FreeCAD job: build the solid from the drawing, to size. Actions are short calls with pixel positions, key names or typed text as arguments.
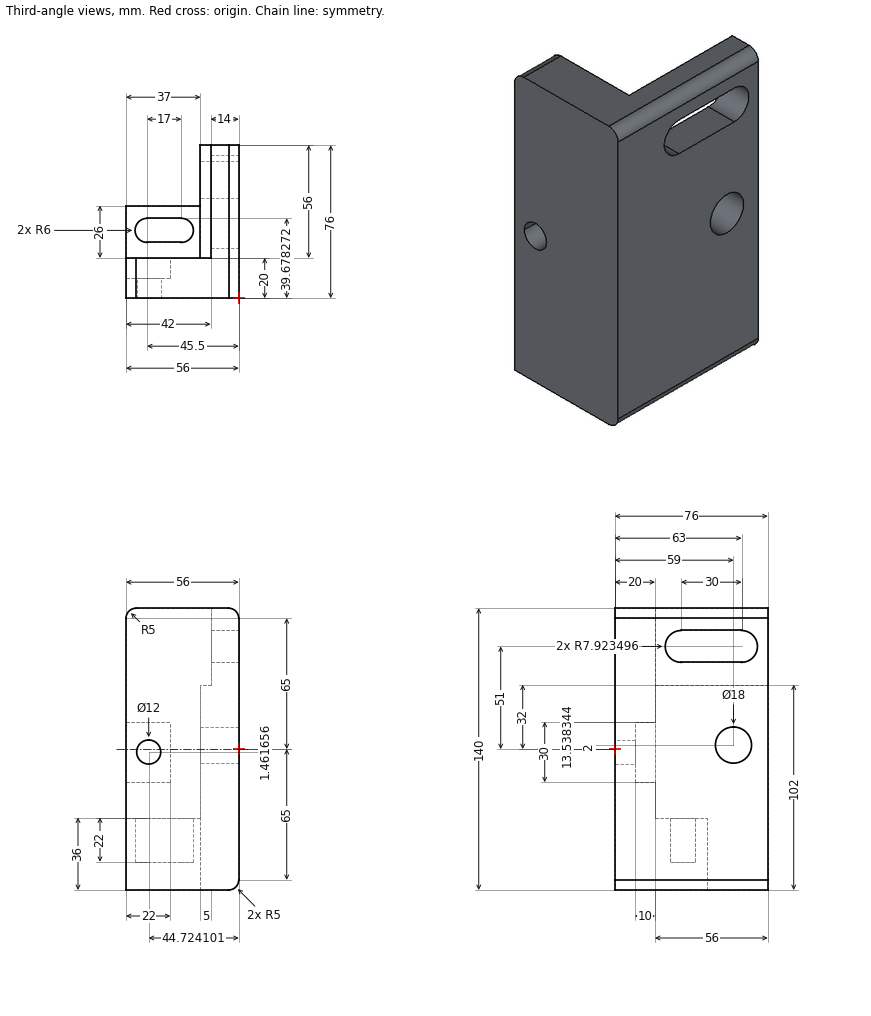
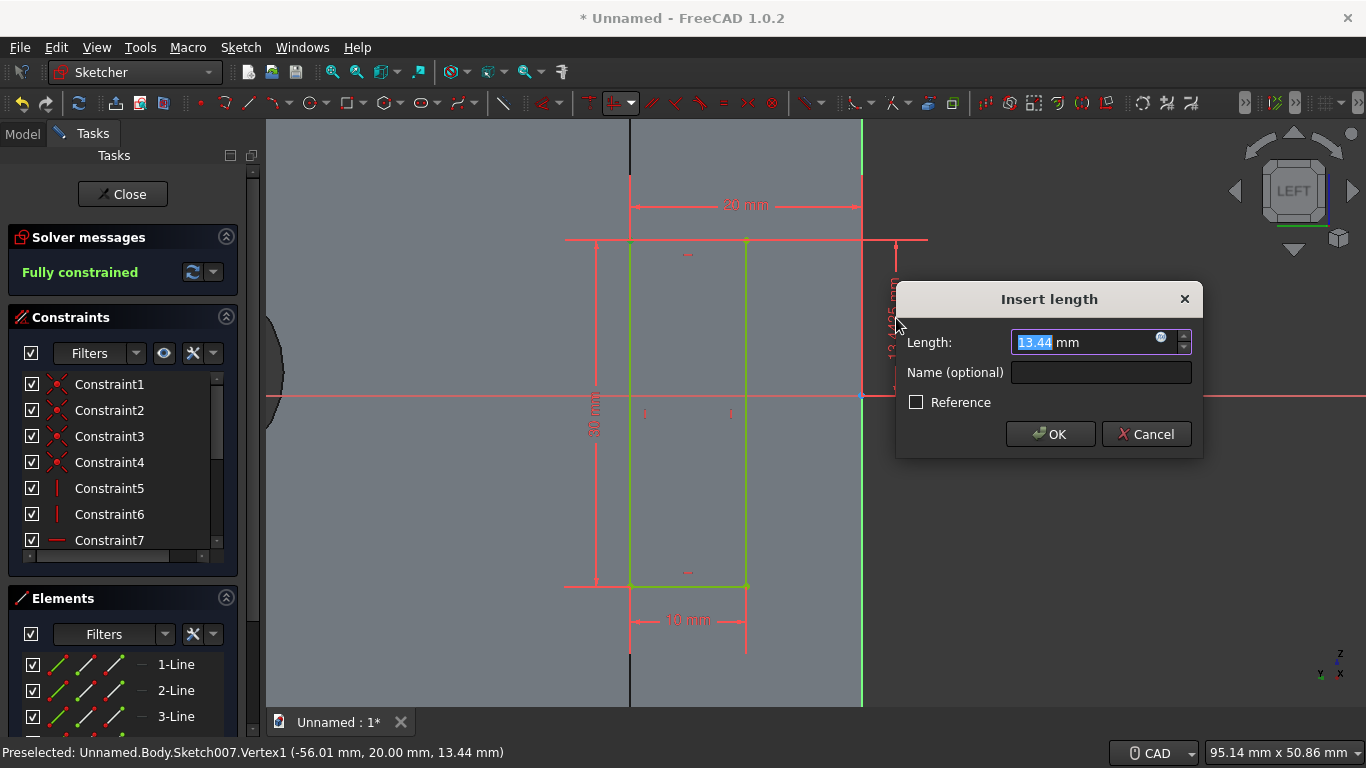
text(13.538344)
key(Return)
key(Escape)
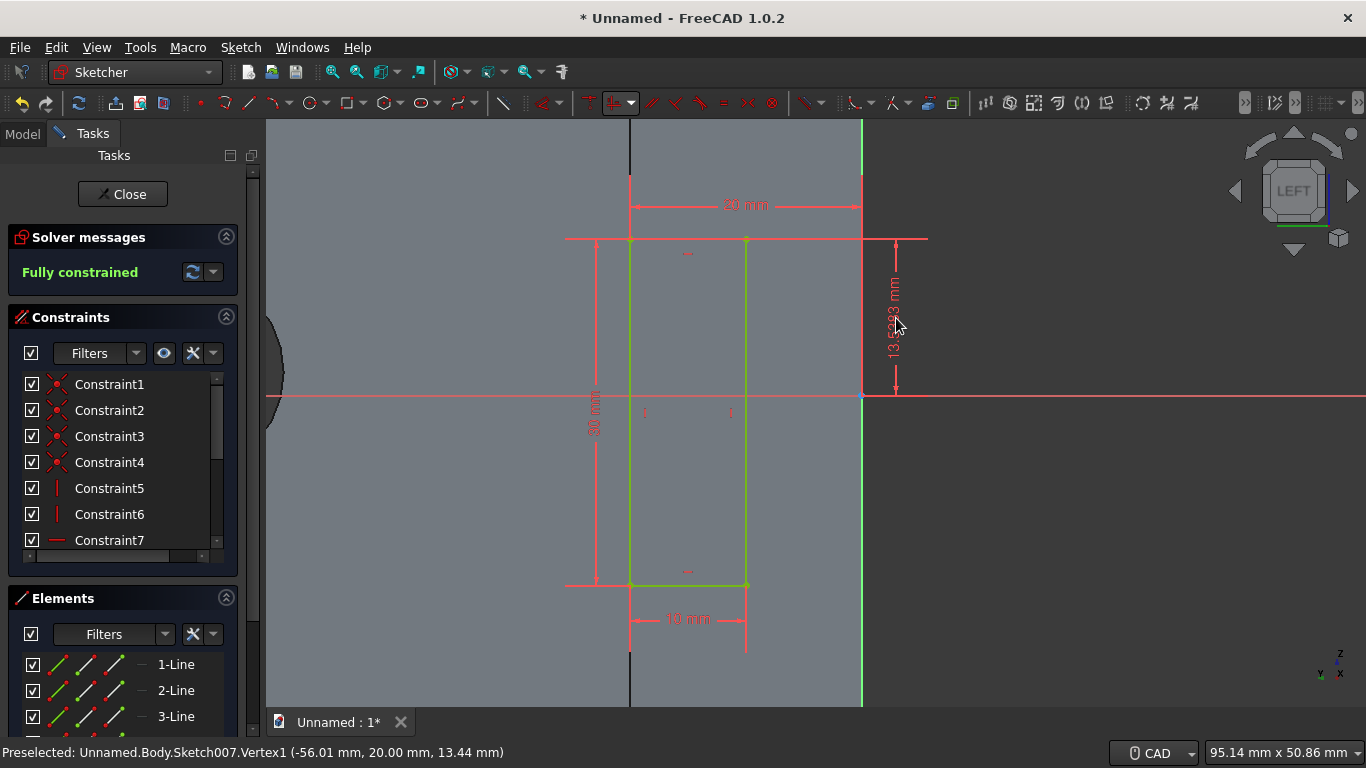
click(123, 194)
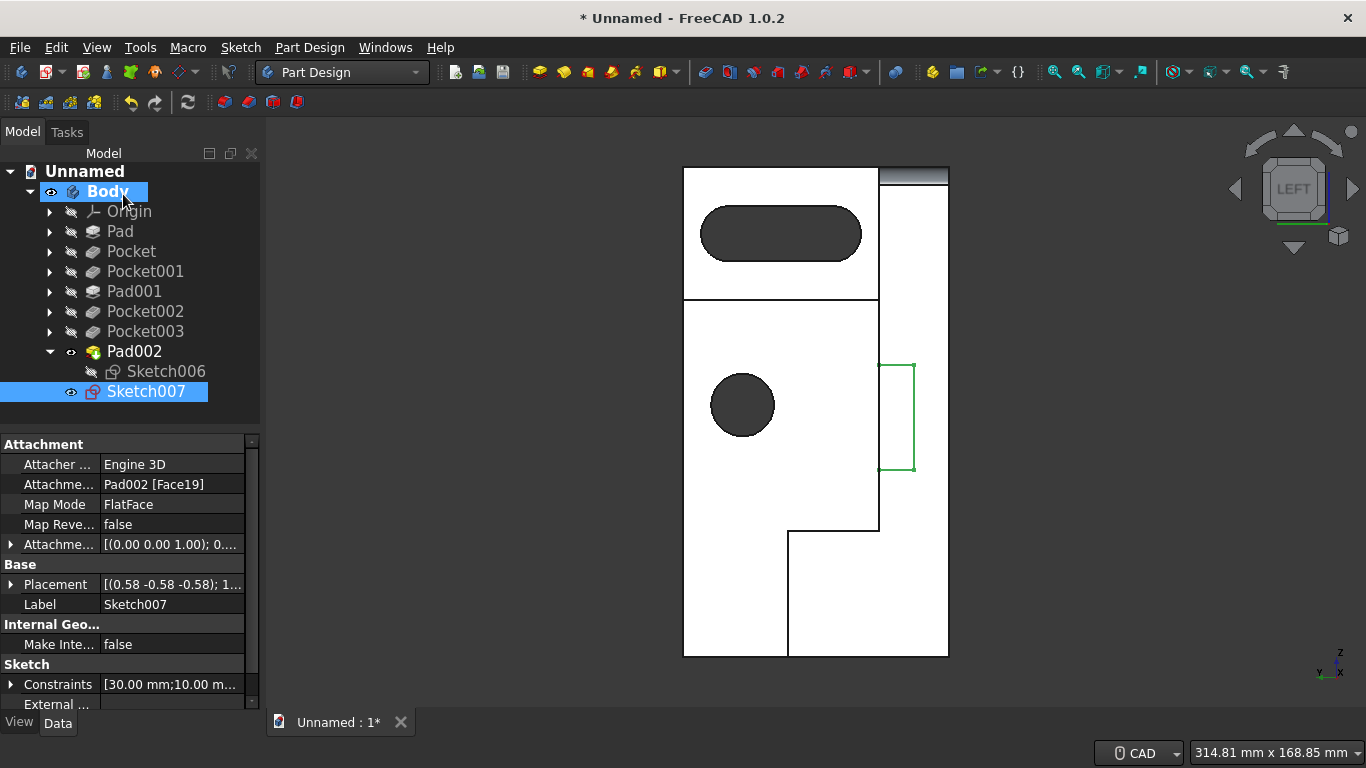
click(706, 72)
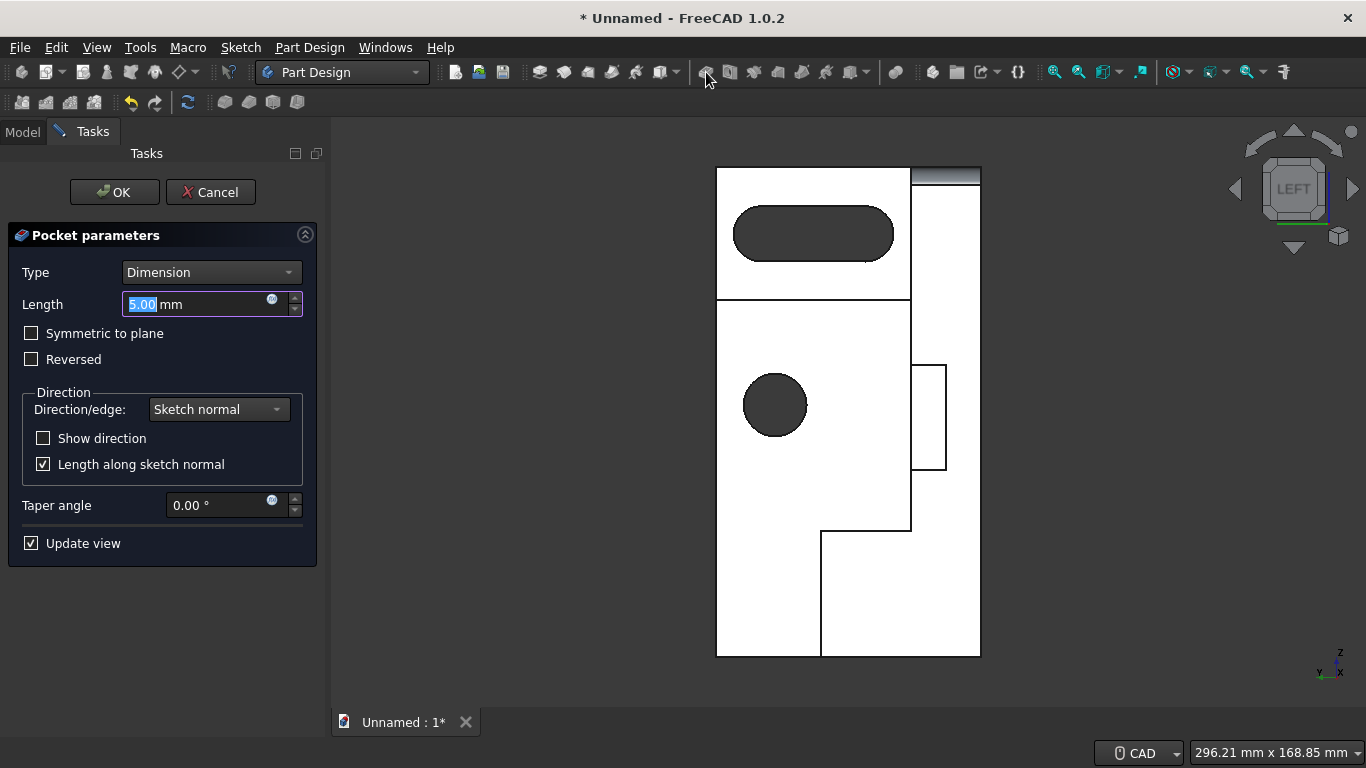
text(22)
key(Tab)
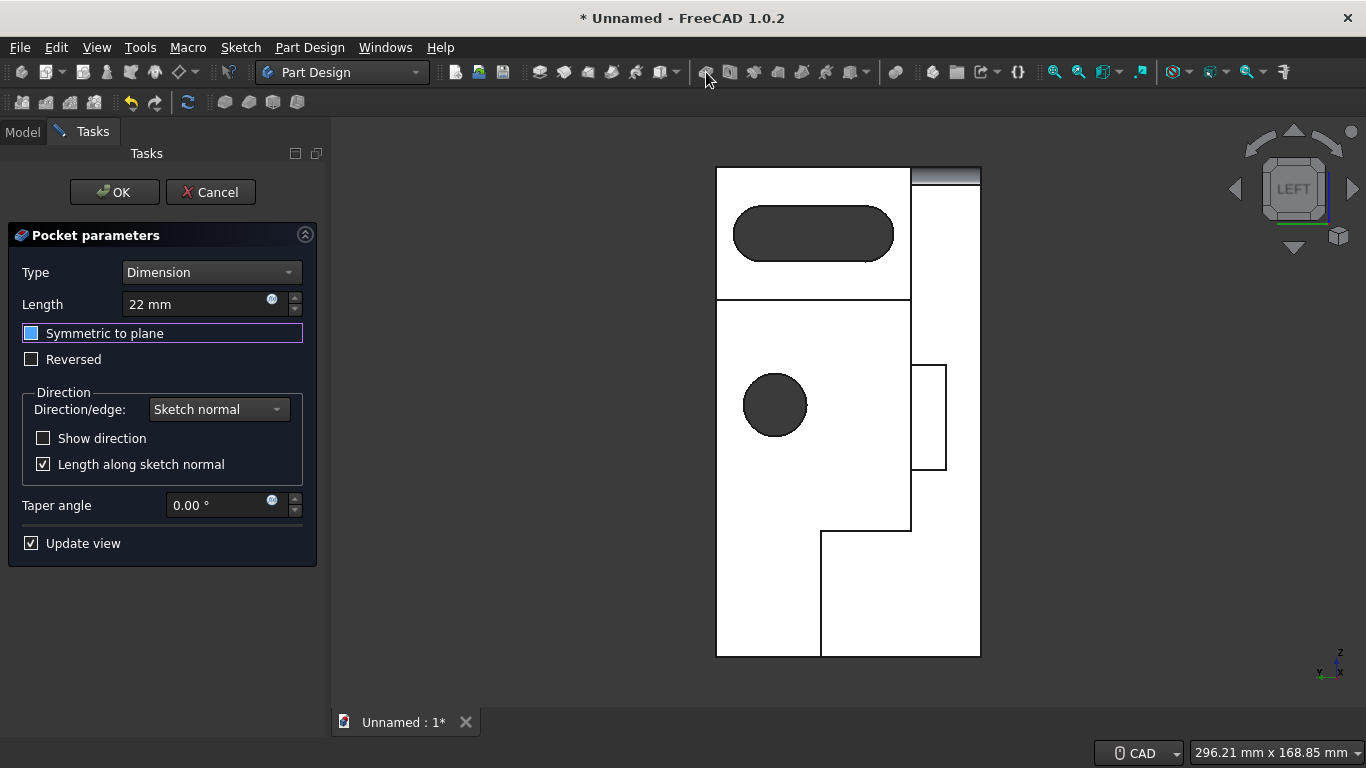
click(115, 192)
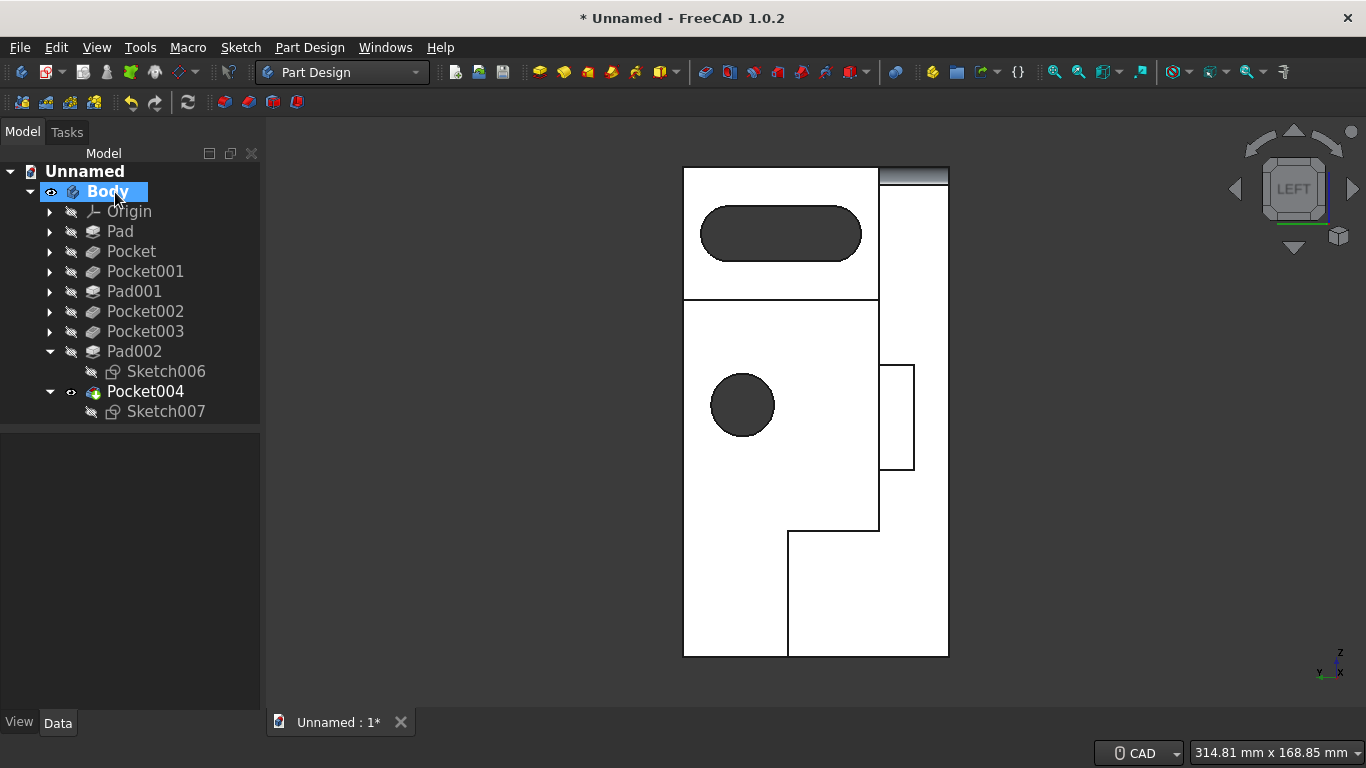
key(4)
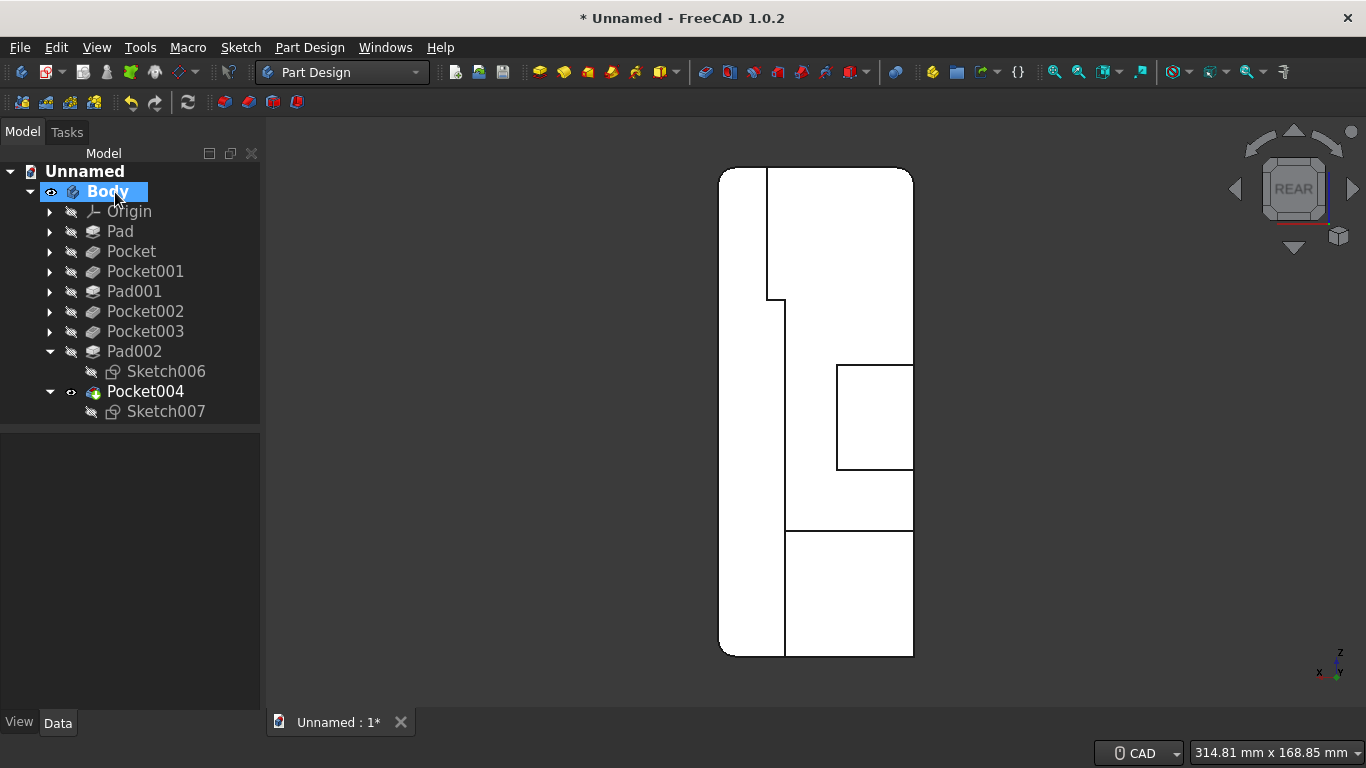
click(875, 416)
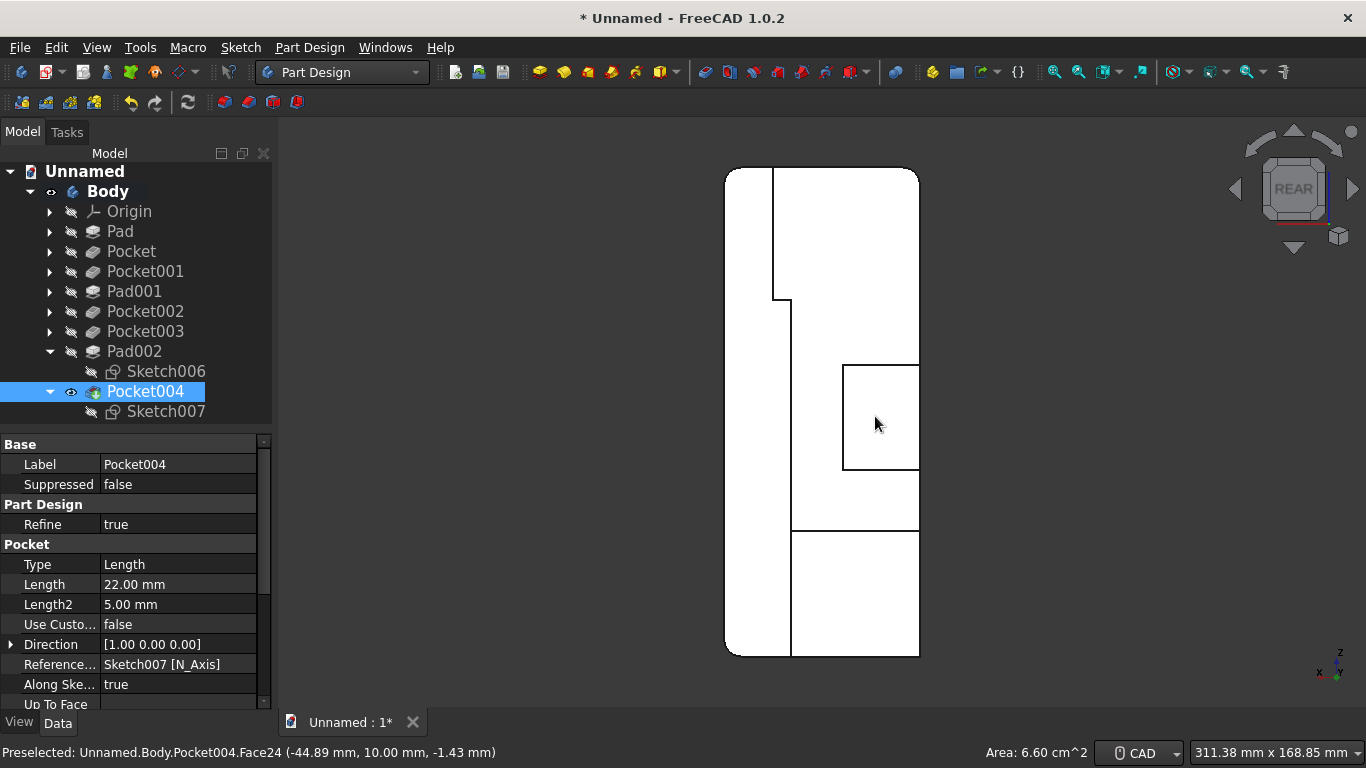
click(46, 72)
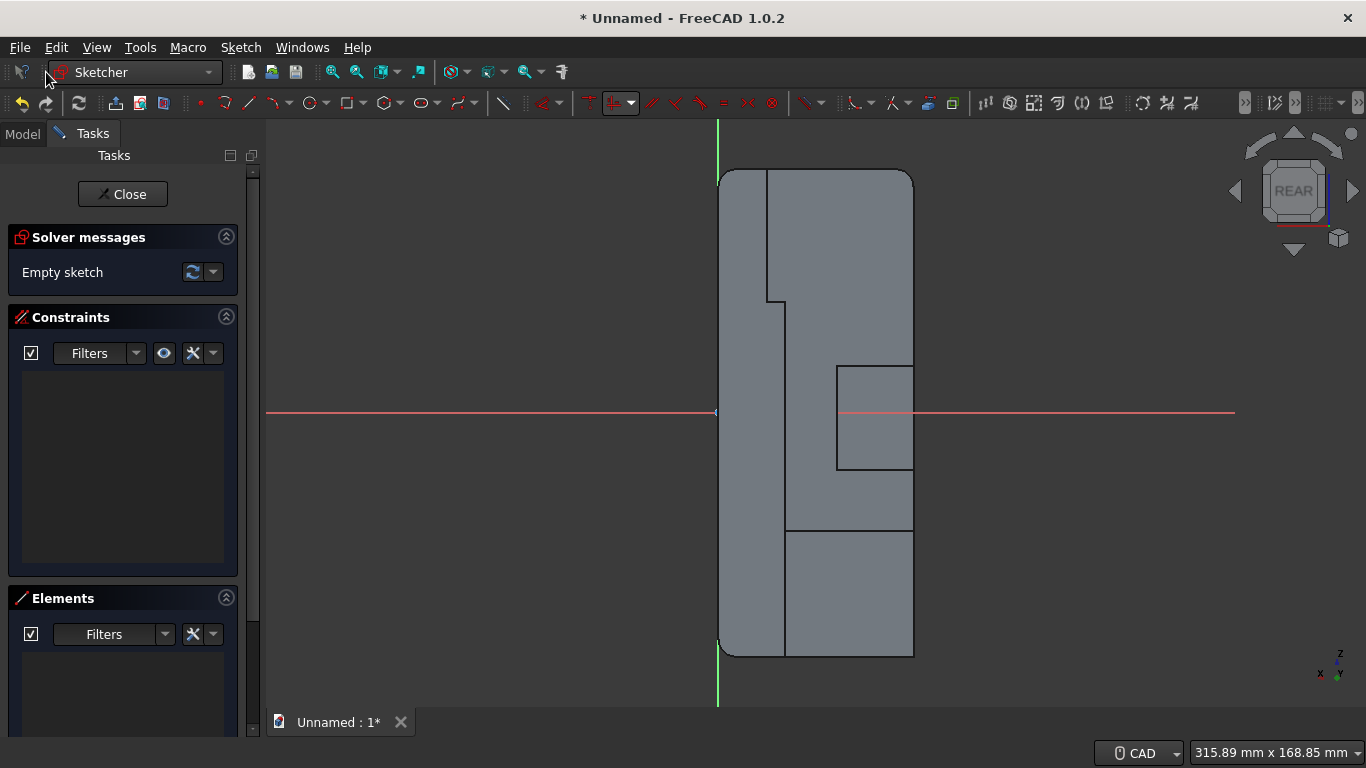
scroll(890, 419, up, 11)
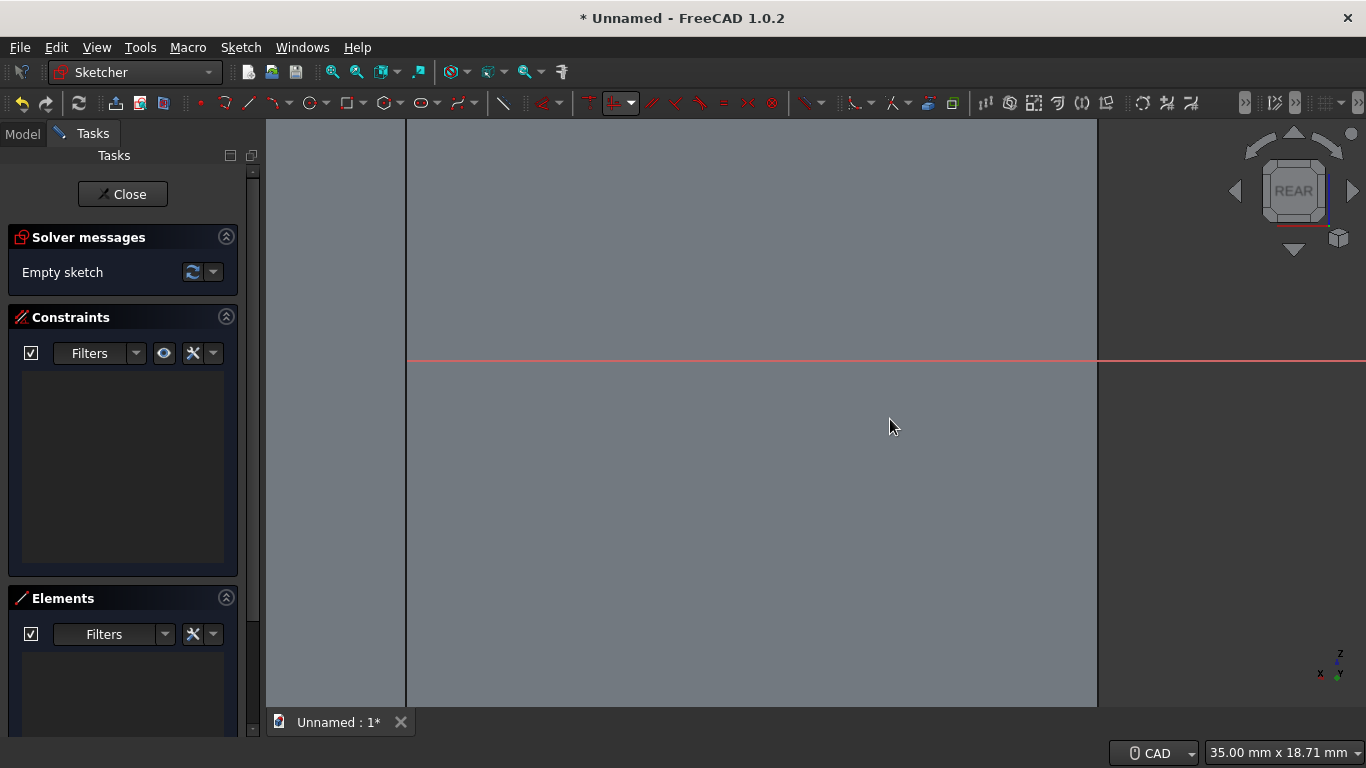
key(g)
key(c)